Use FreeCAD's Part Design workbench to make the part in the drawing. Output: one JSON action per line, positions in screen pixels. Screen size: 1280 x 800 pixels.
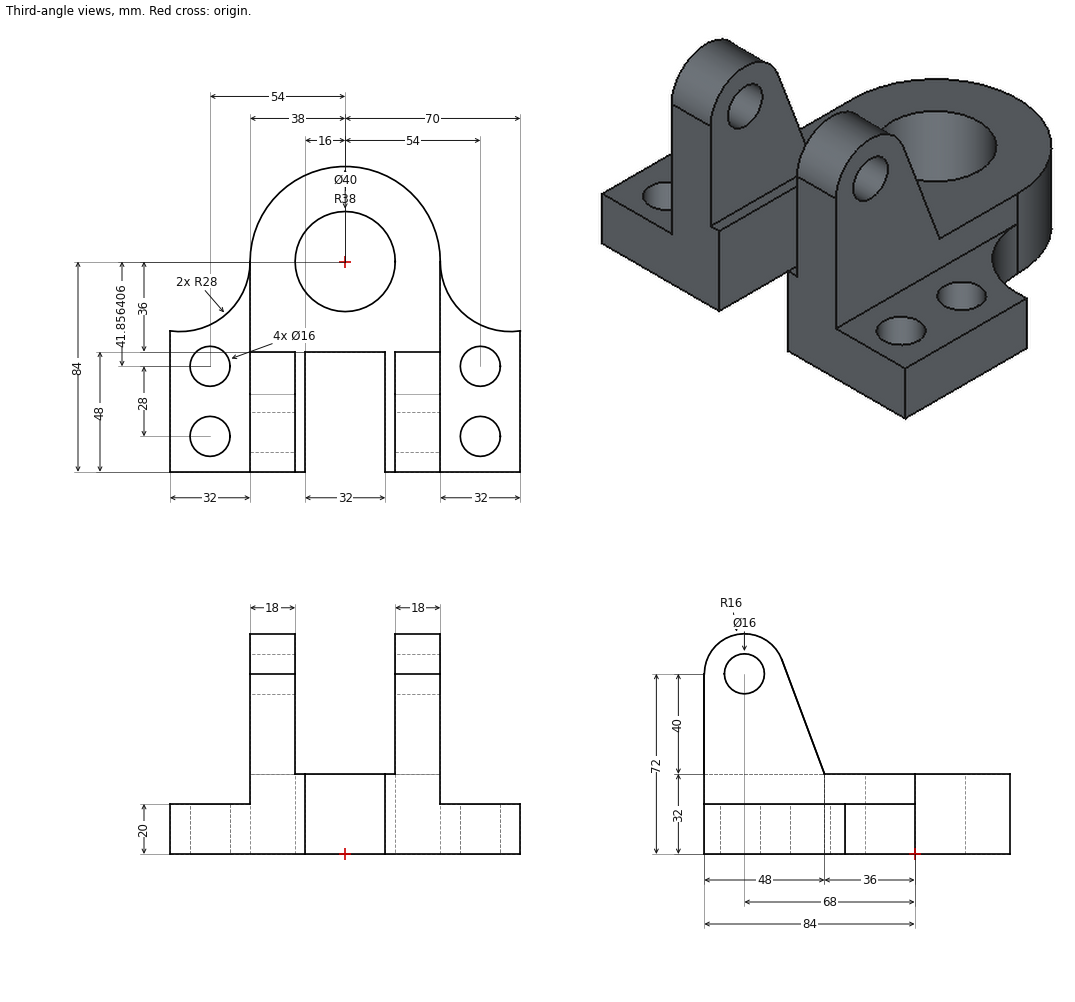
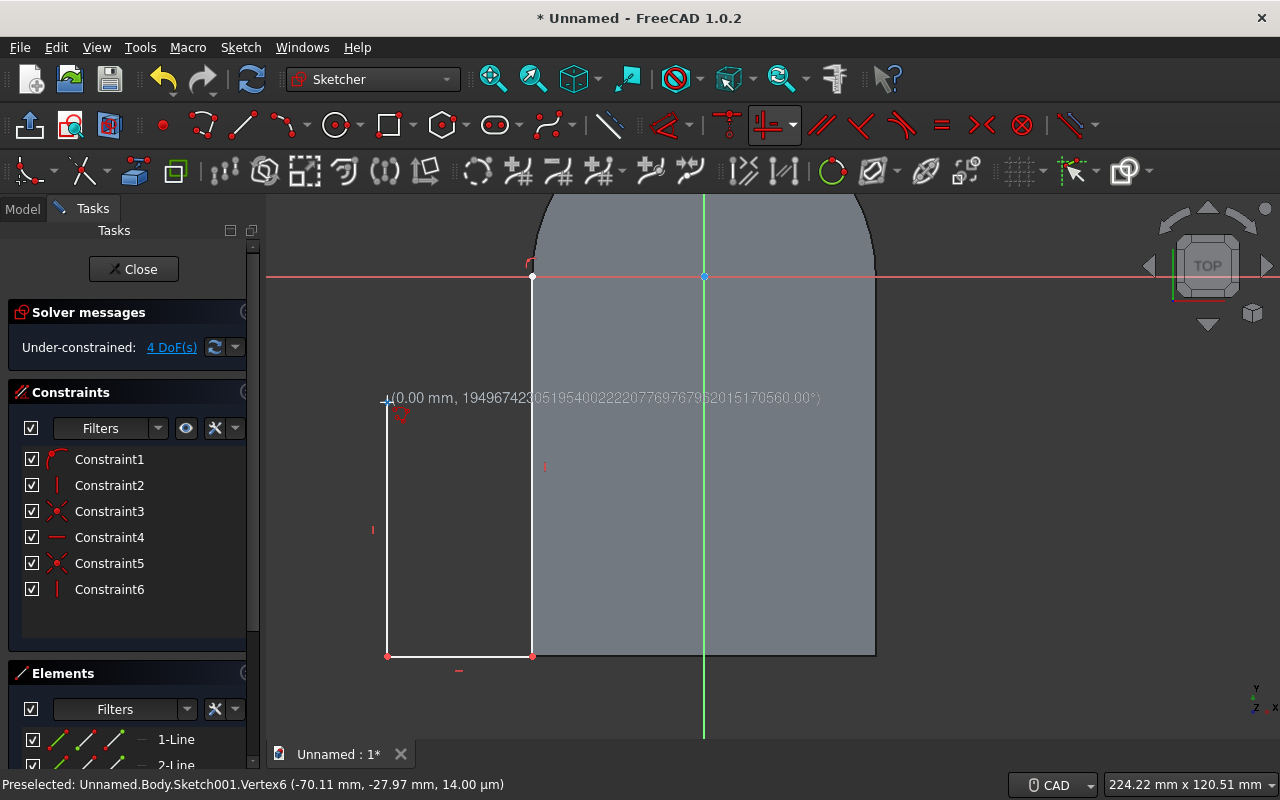
{"action": "left_click", "coordinate": [284, 126]}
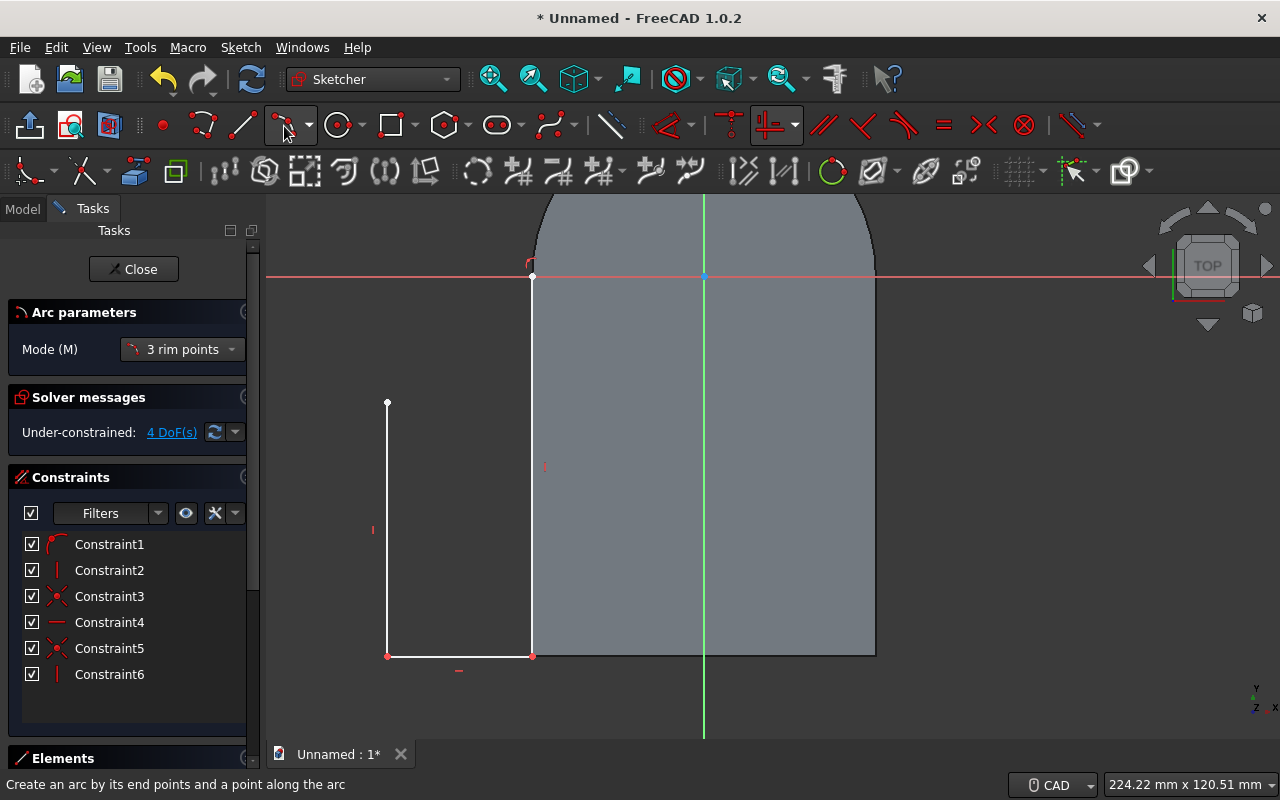
{"action": "left_click", "coordinate": [387, 403]}
{"action": "left_click", "coordinate": [532, 277]}
{"action": "left_click", "coordinate": [488, 372]}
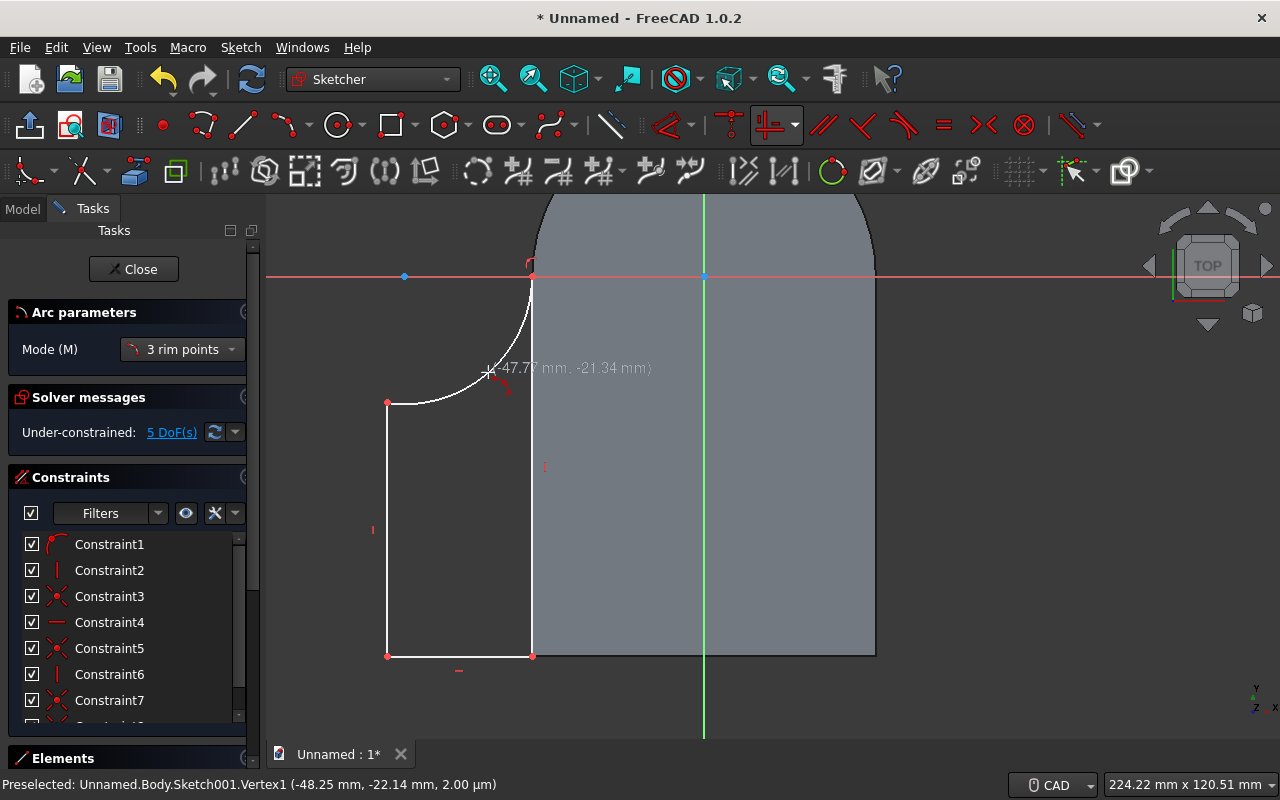
{"action": "left_click", "coordinate": [204, 126]}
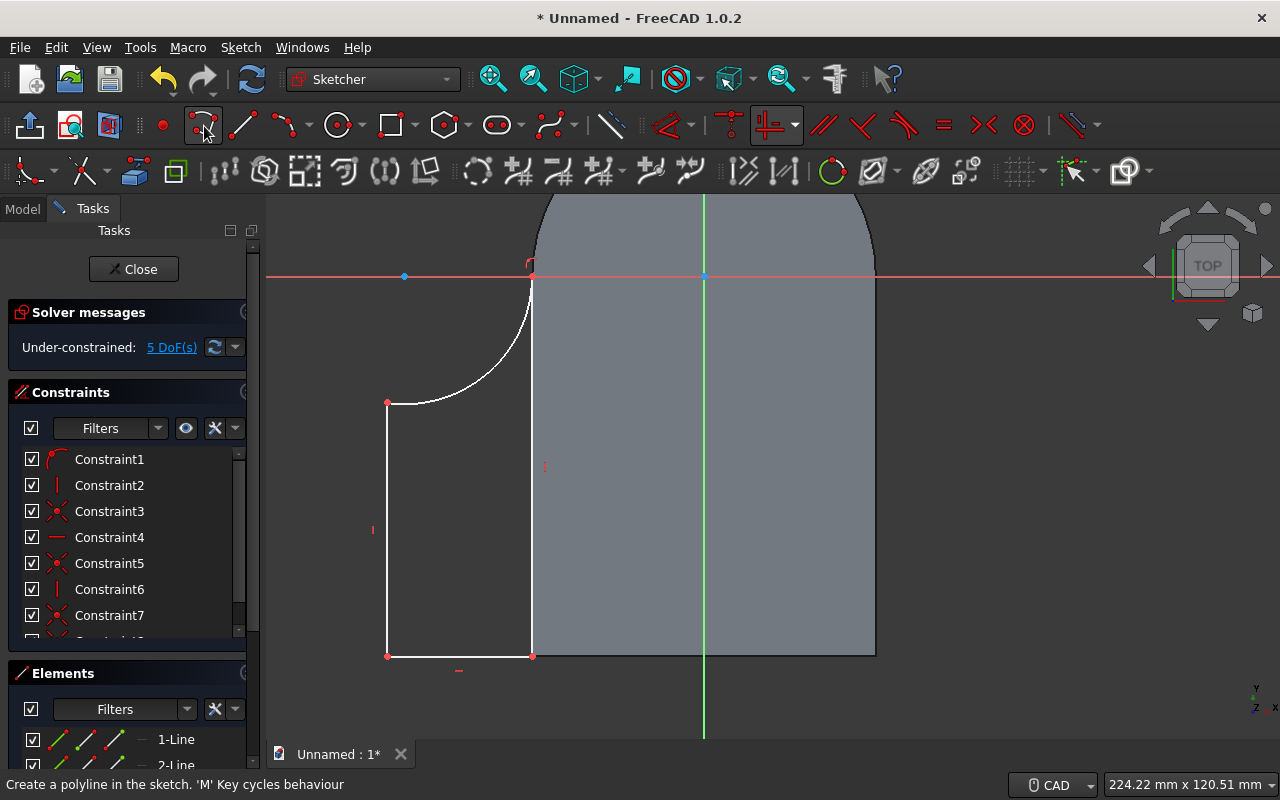
{"action": "left_click", "coordinate": [1021, 402]}
{"action": "left_click", "coordinate": [1021, 656]}
{"action": "left_click", "coordinate": [876, 656]}
{"action": "left_click", "coordinate": [876, 277]}
{"action": "right_click", "coordinate": [876, 277]}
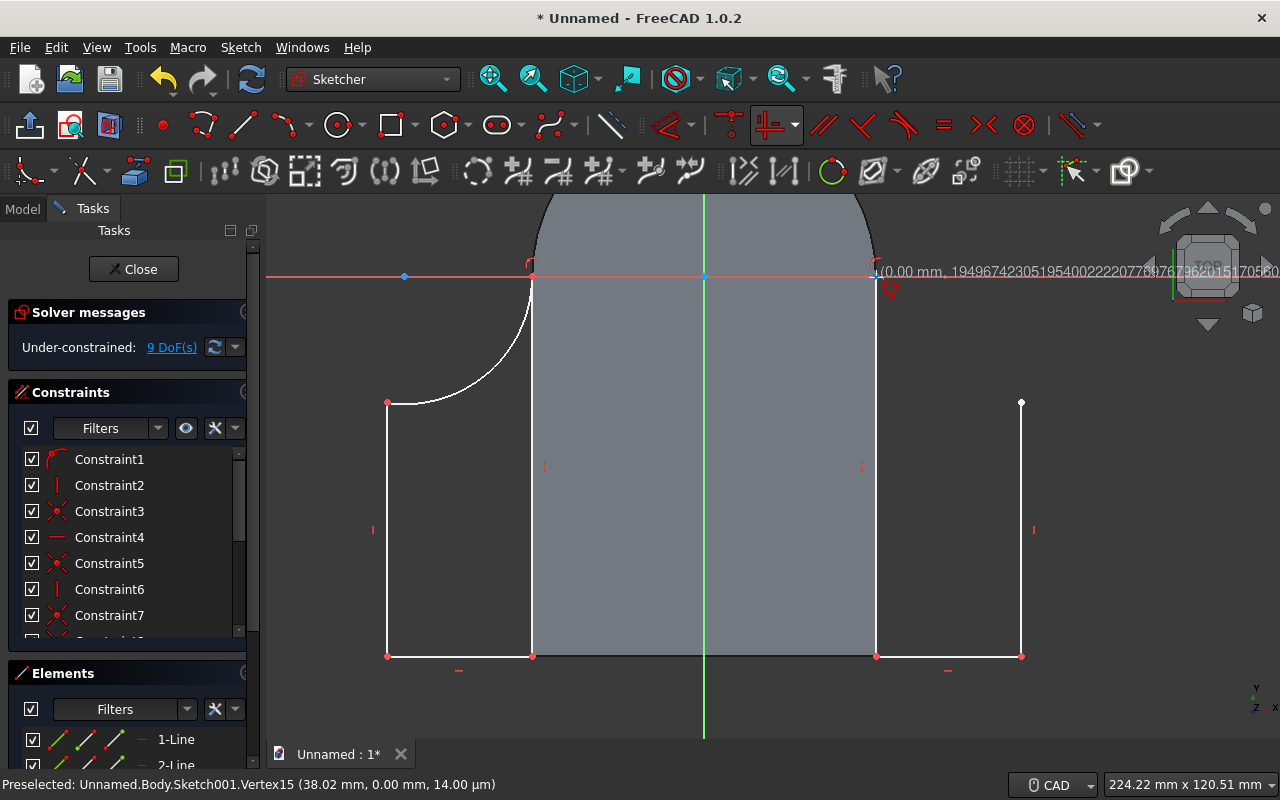
{"action": "left_click", "coordinate": [284, 126]}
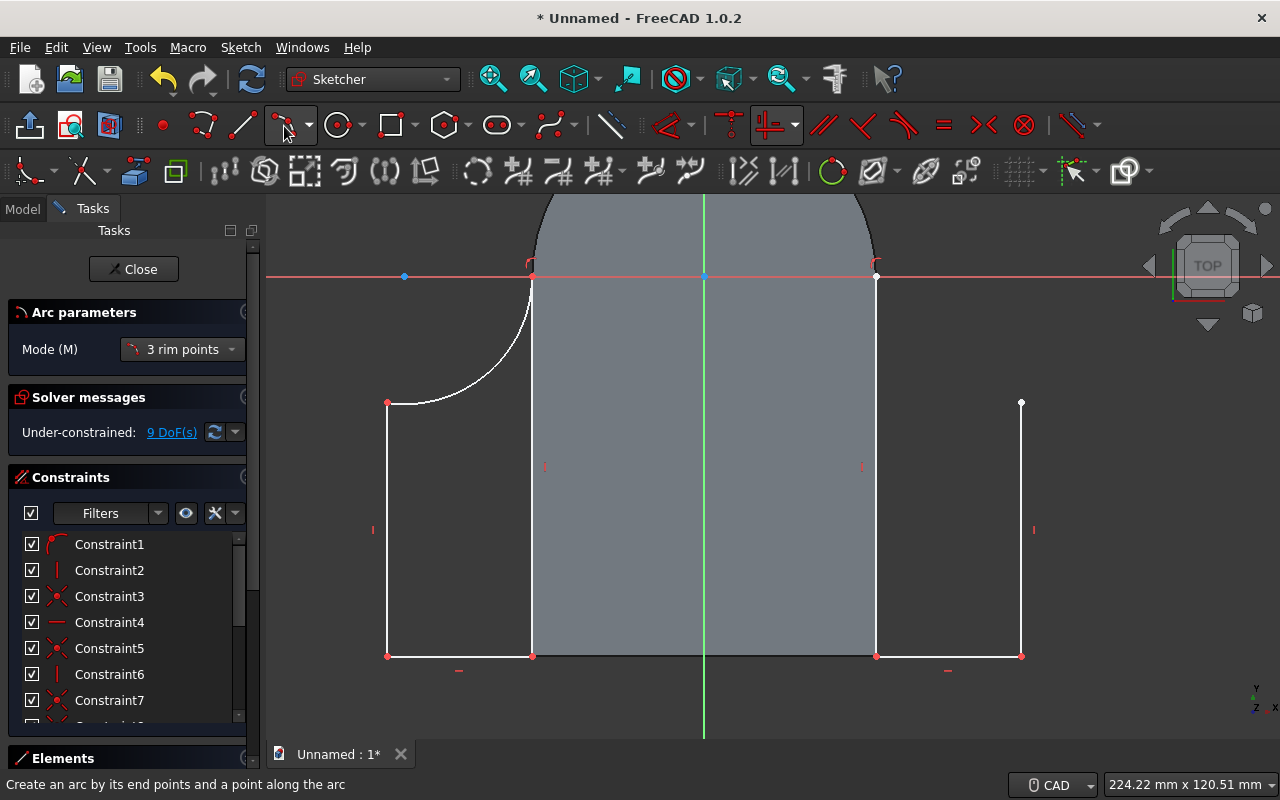
{"action": "left_click", "coordinate": [876, 277]}
{"action": "left_click", "coordinate": [1021, 403]}
{"action": "left_click", "coordinate": [920, 372]}
{"action": "key", "text": "Escape"}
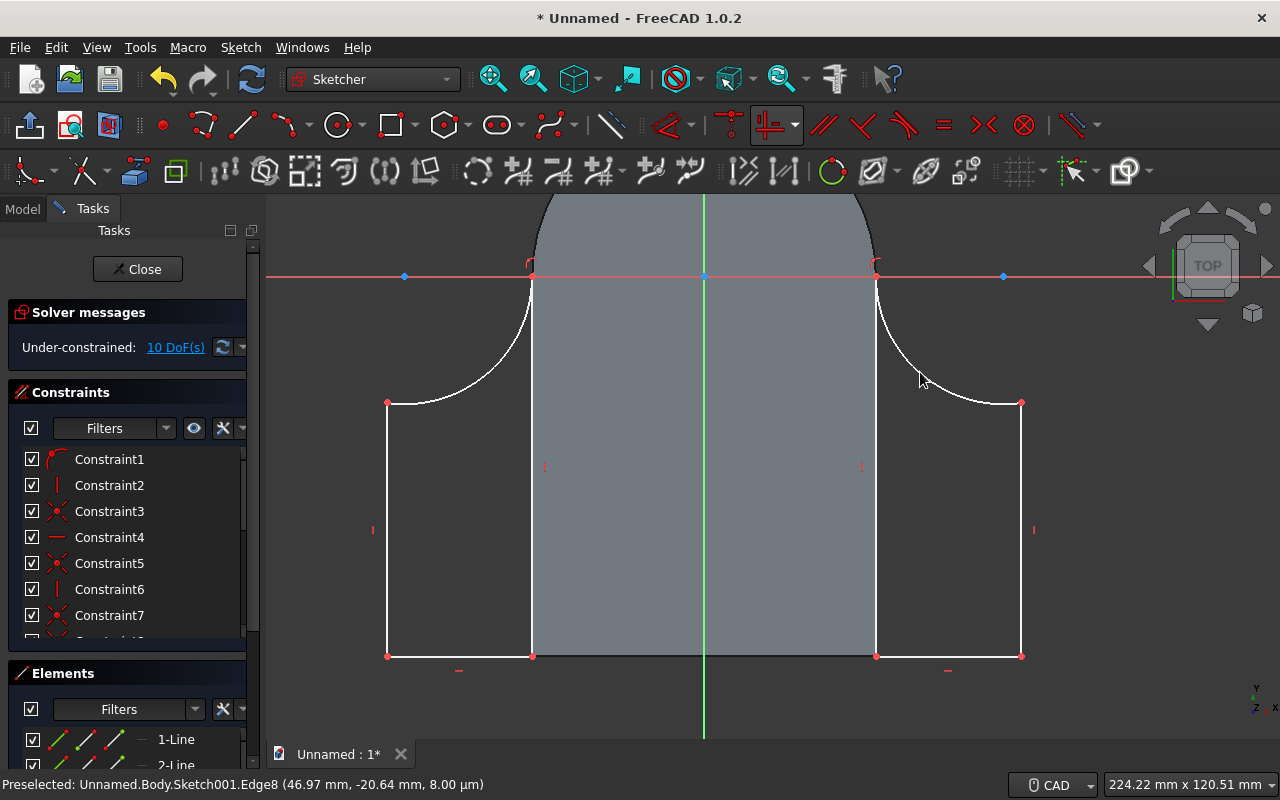
{"action": "left_click", "coordinate": [532, 391]}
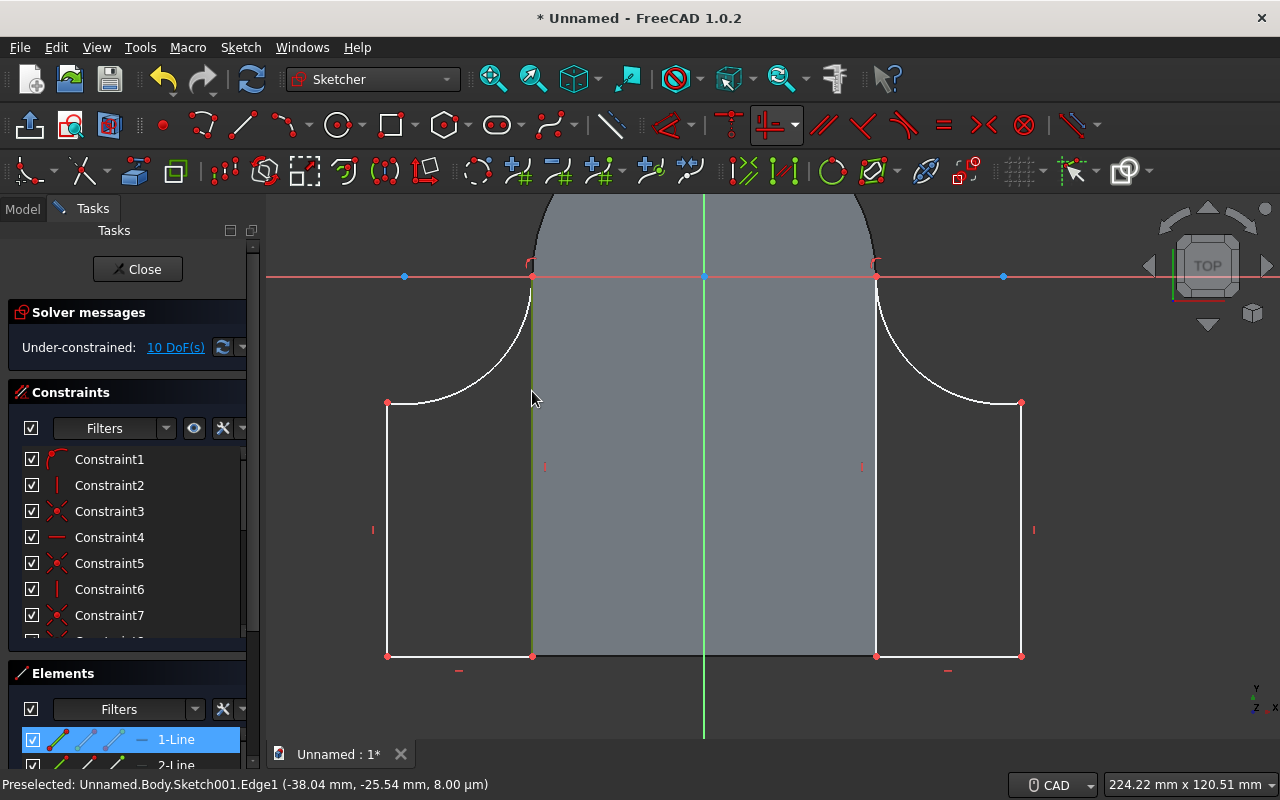
{"action": "left_click", "coordinate": [451, 395]}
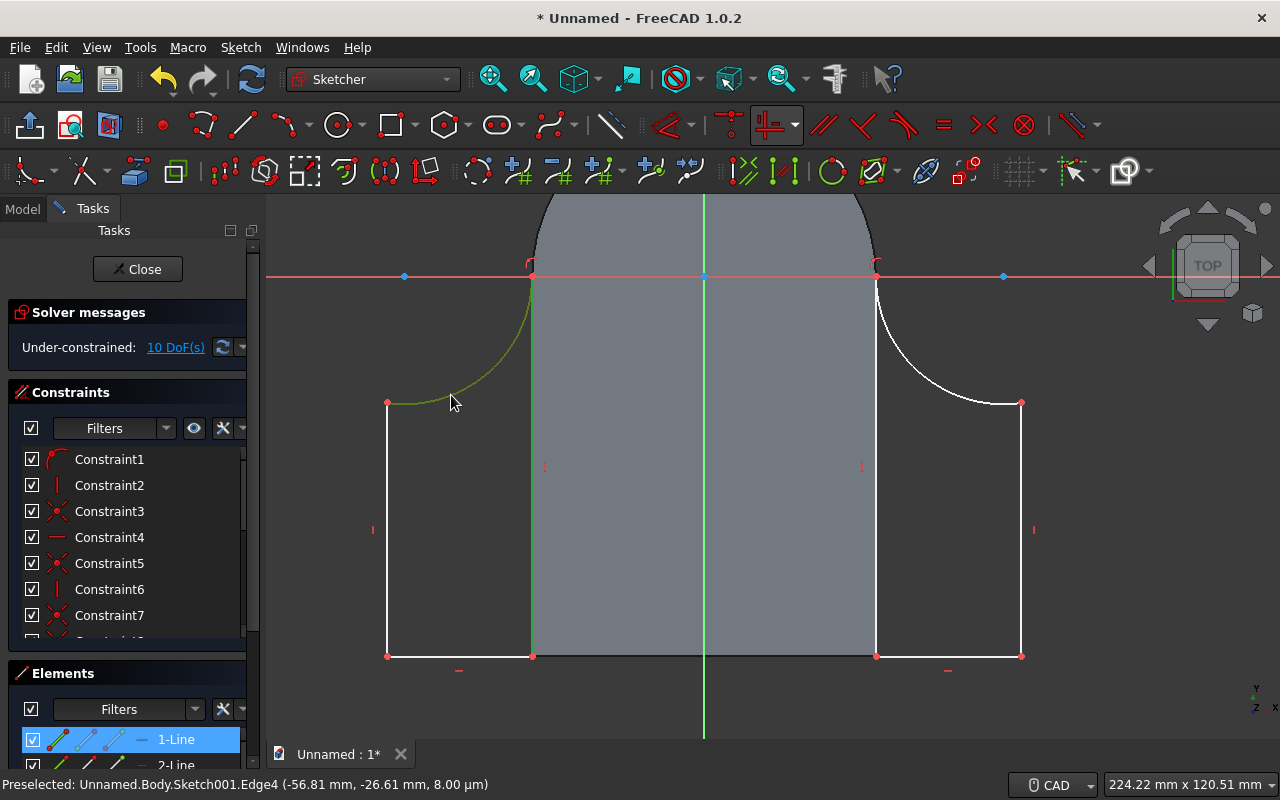
{"action": "left_click", "coordinate": [904, 126]}